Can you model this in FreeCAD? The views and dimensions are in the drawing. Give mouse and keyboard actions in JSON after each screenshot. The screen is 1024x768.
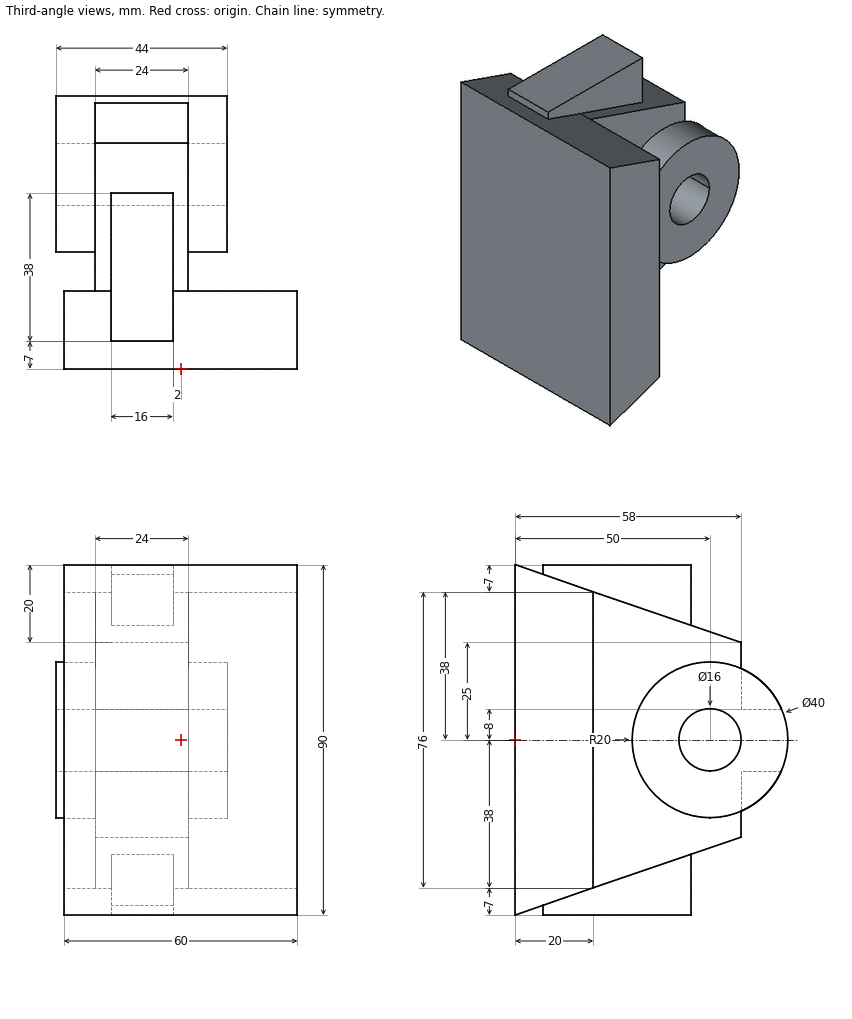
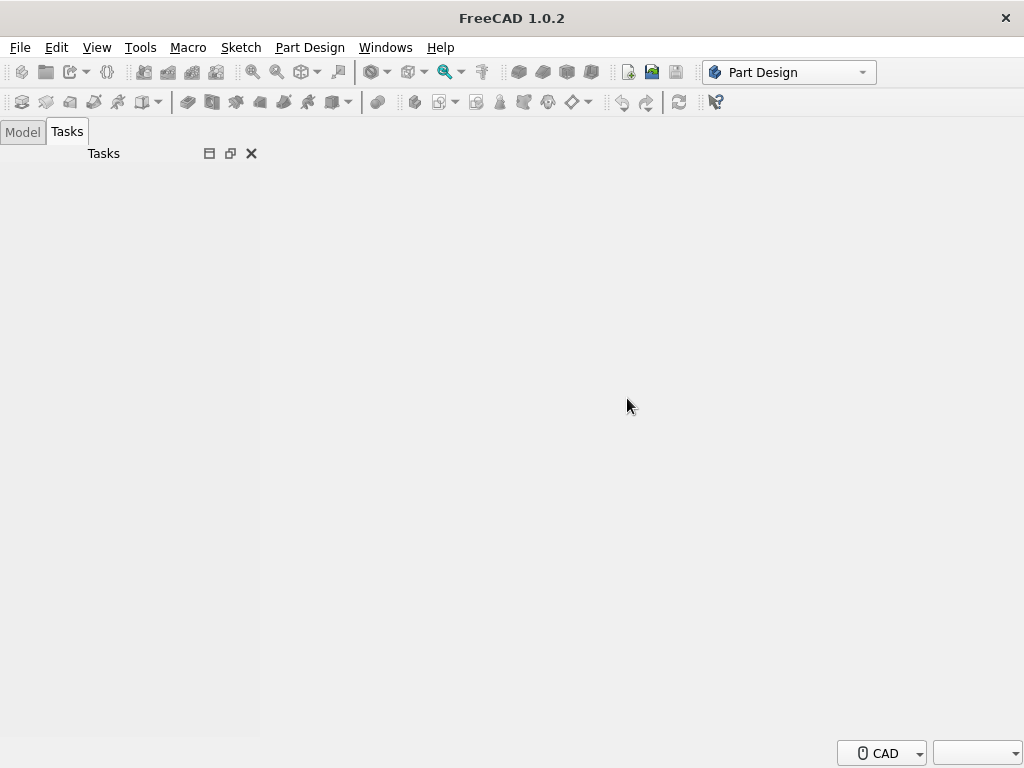
{"action": "left_click", "coordinate": [628, 72]}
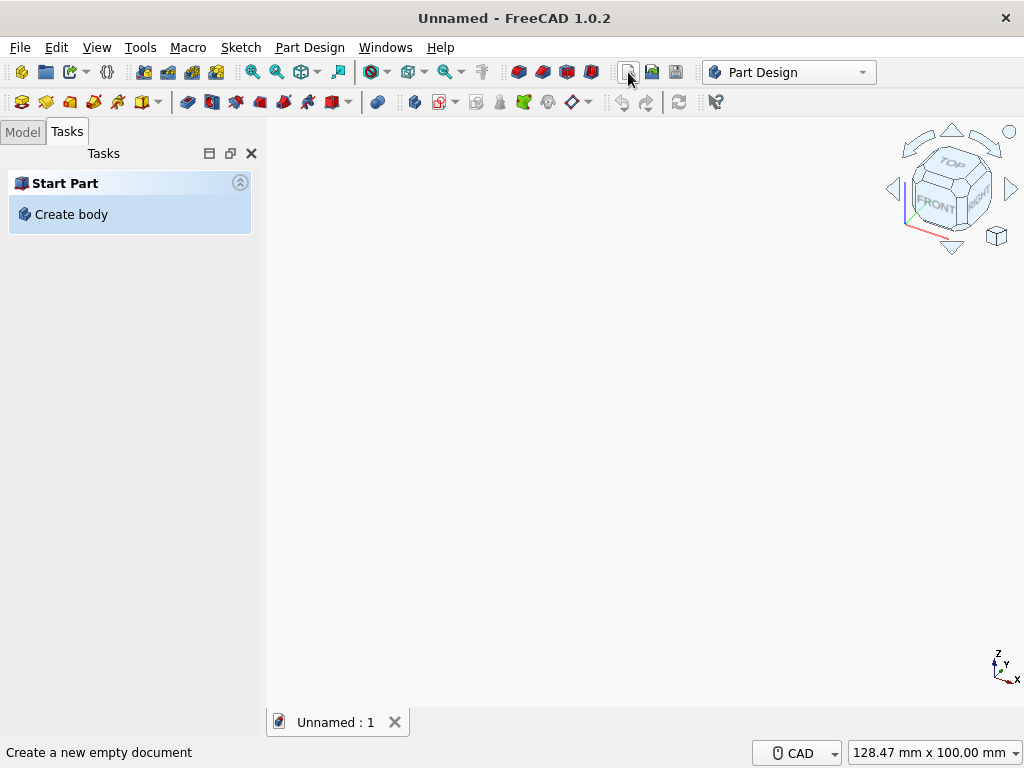
{"action": "left_click", "coordinate": [440, 102]}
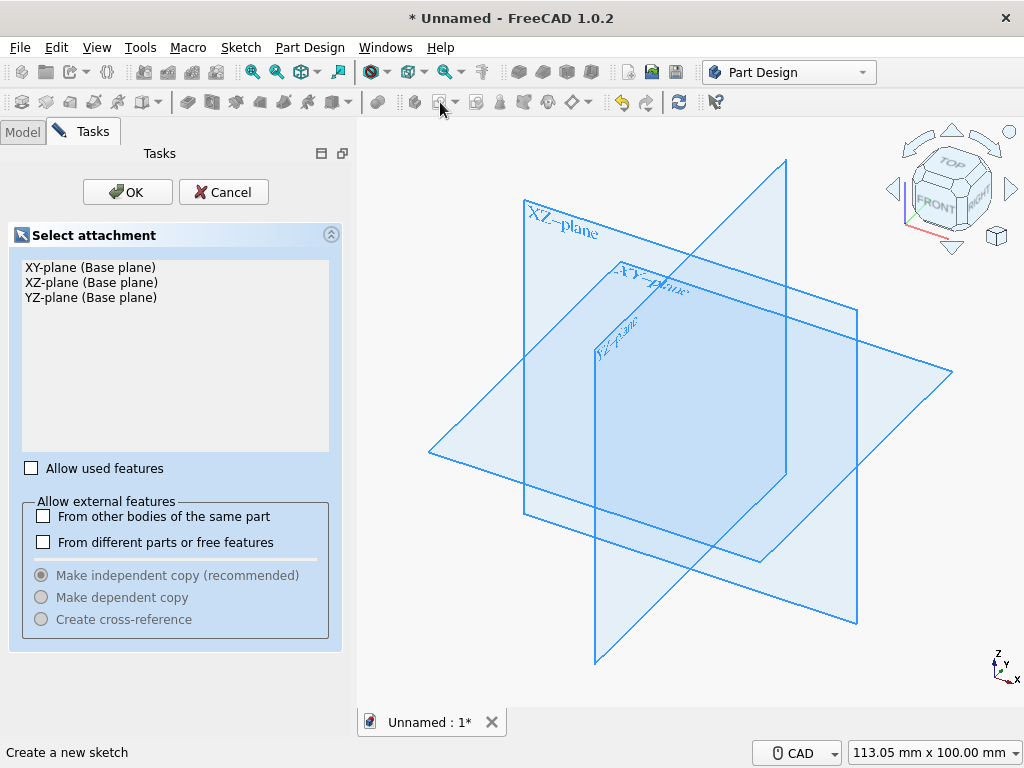
{"action": "left_click", "coordinate": [82, 282]}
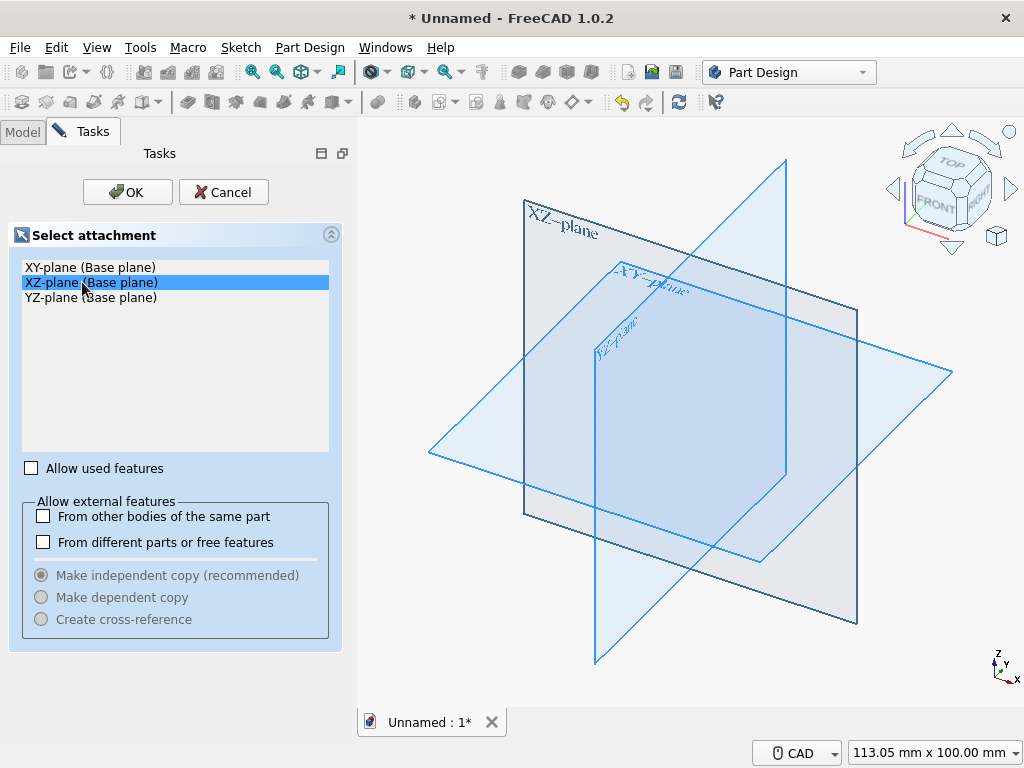
{"action": "left_click", "coordinate": [128, 192]}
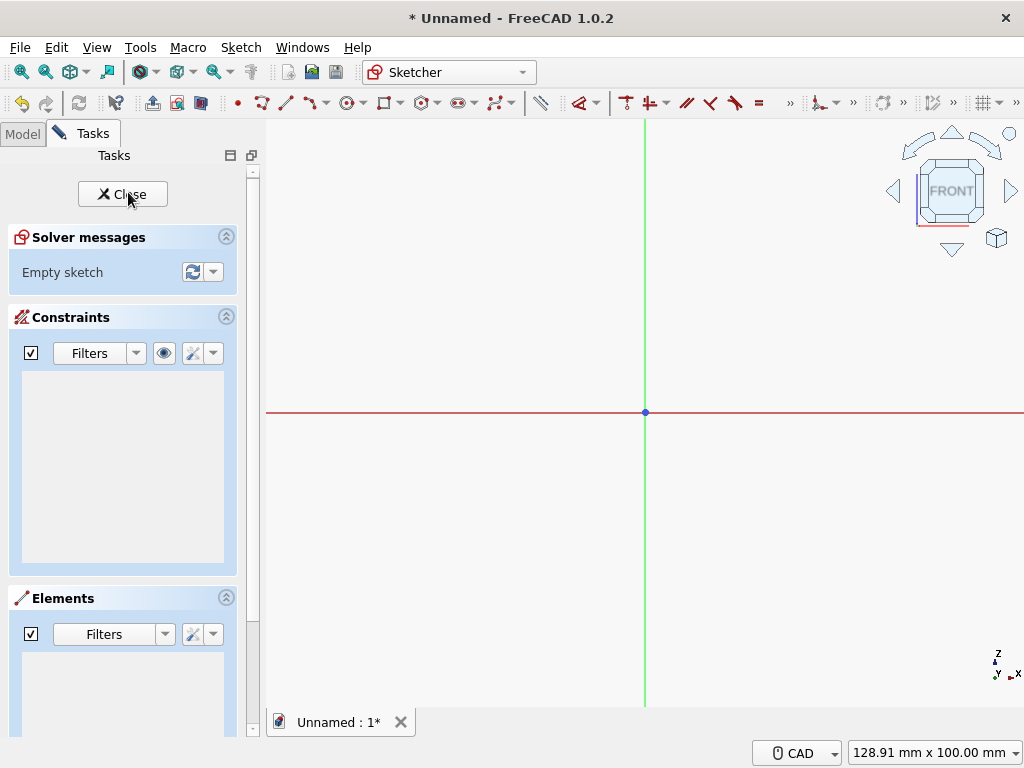
{"action": "scroll", "coordinate": [437, 413], "scroll_direction": "down", "scroll_amount": 2}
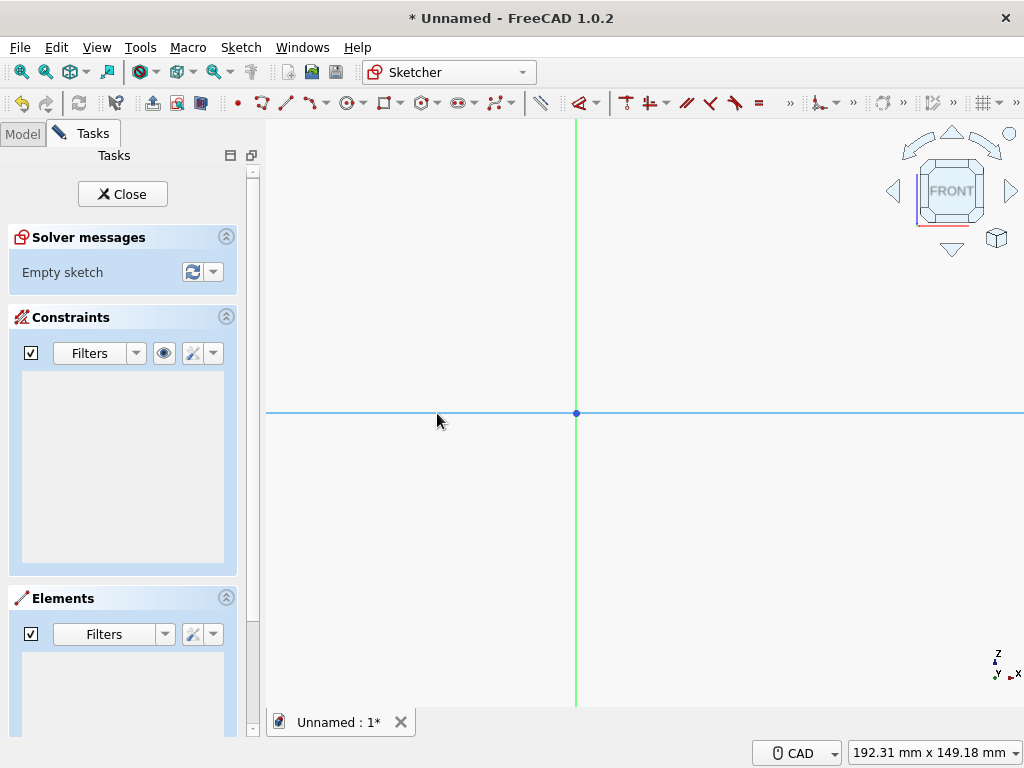
{"action": "key", "text": "g v"}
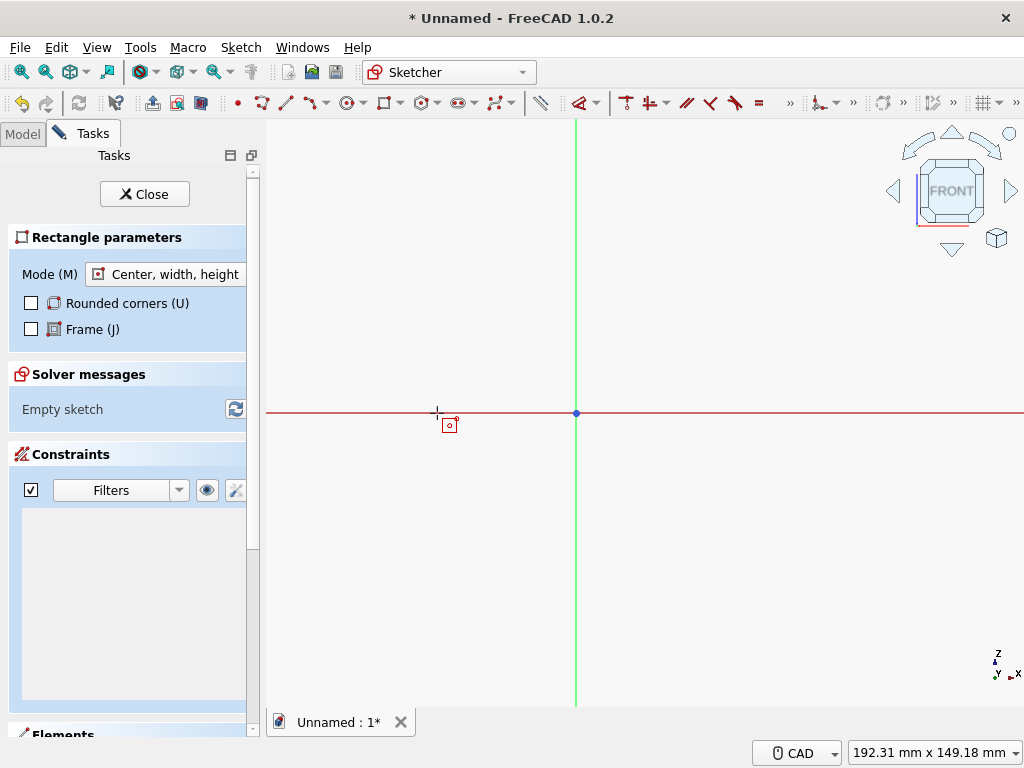
{"action": "left_click", "coordinate": [577, 413]}
{"action": "mouse_move", "coordinate": [695, 236]}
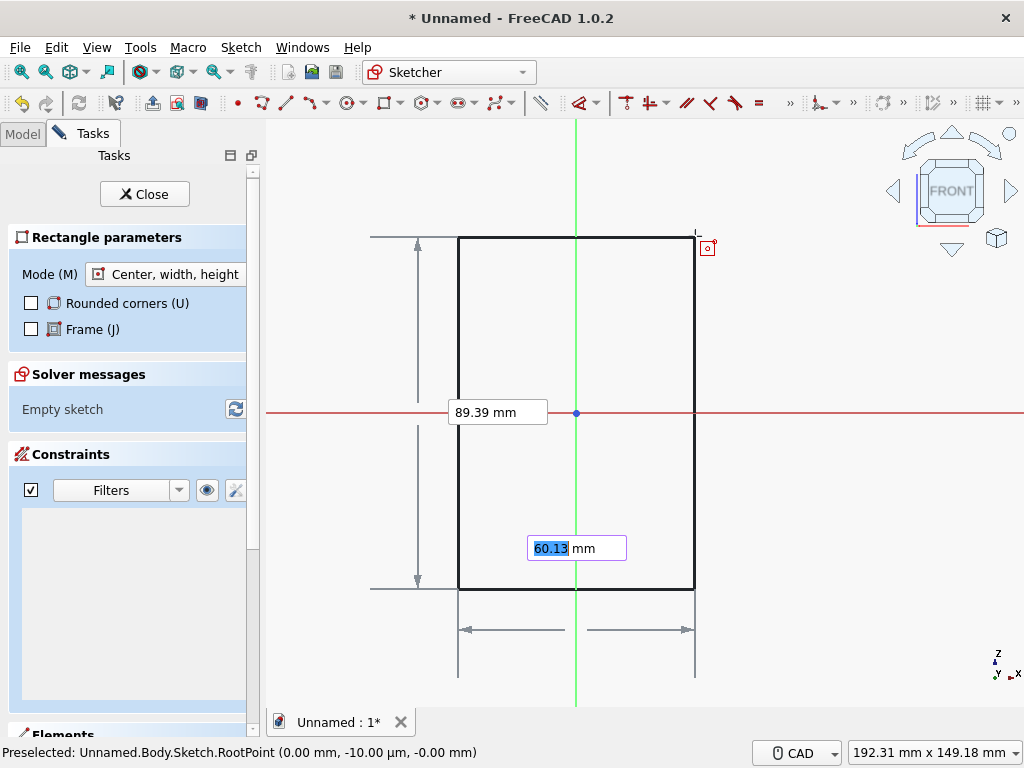
{"action": "type", "text": "60"}
{"action": "key", "text": "Tab"}
{"action": "type", "text": "90"}
{"action": "key", "text": "Return"}
{"action": "key", "text": "Escape"}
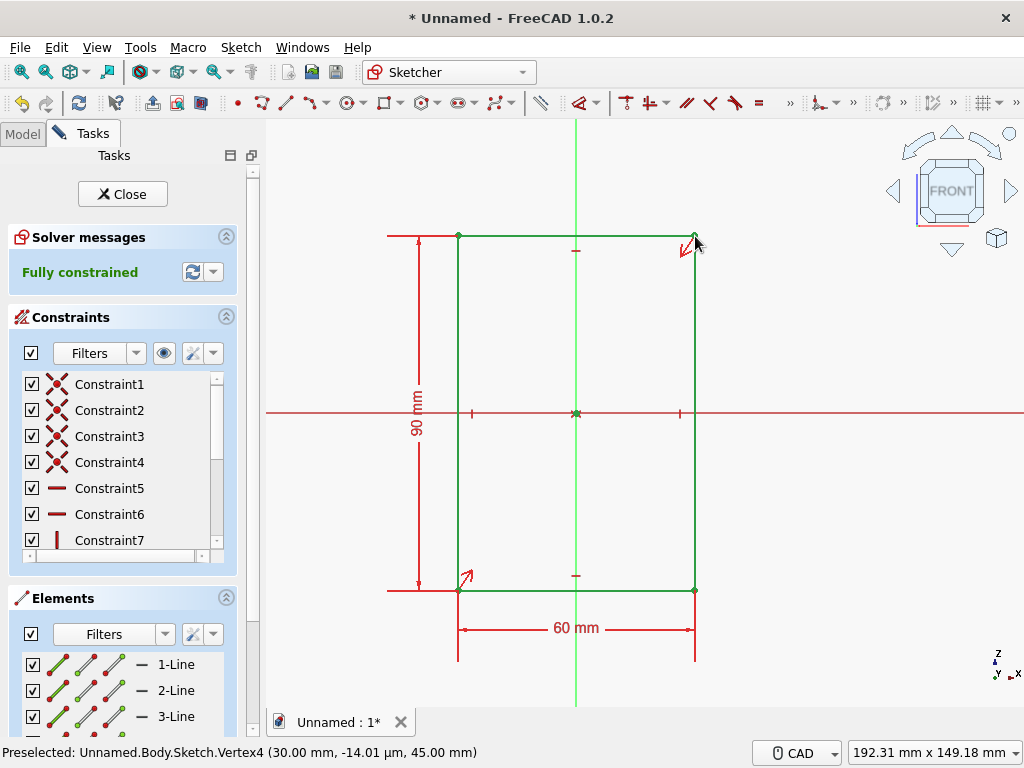
{"action": "left_click", "coordinate": [123, 194]}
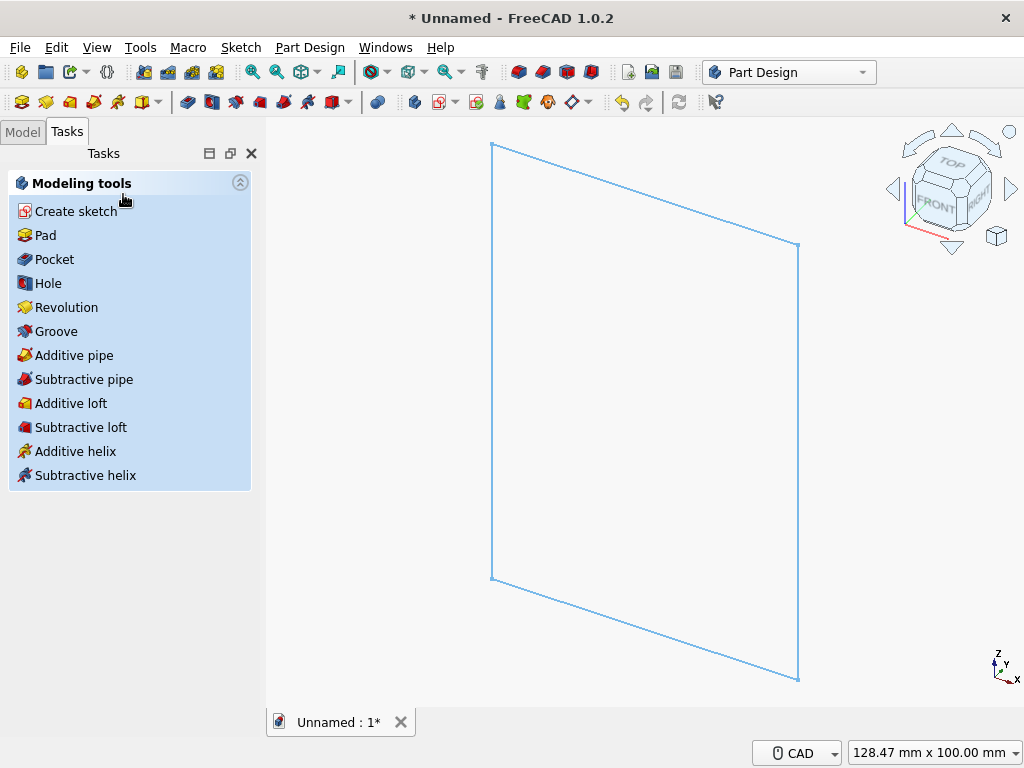
{"action": "left_click", "coordinate": [22, 102]}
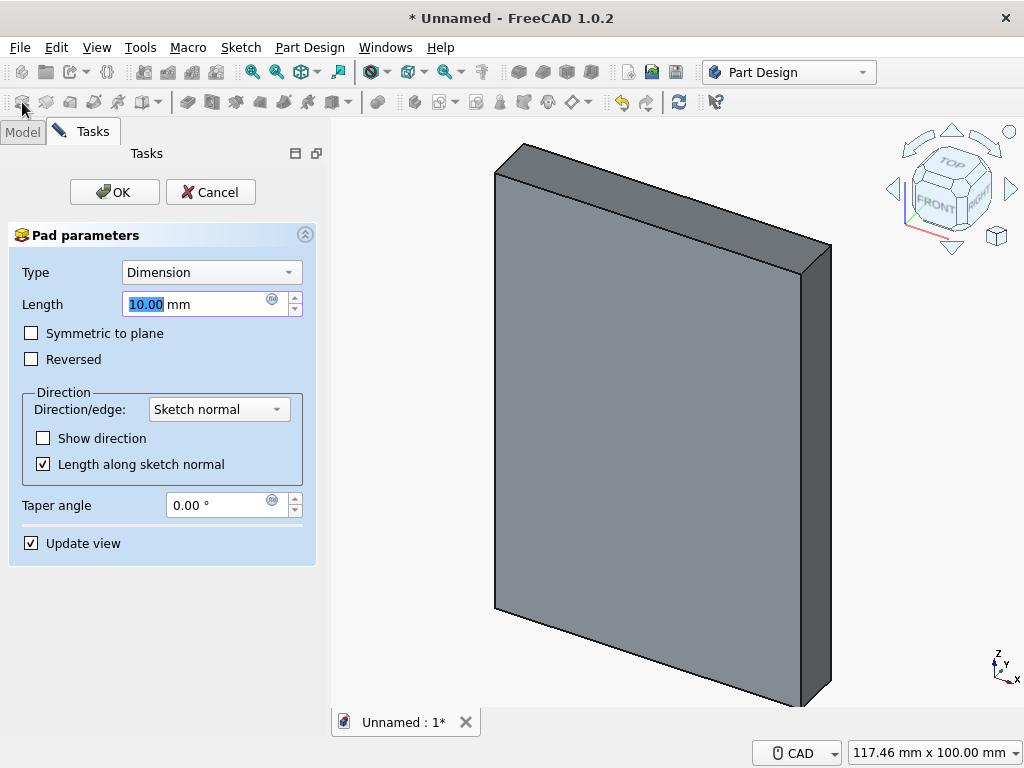
{"action": "type", "text": "20"}
{"action": "key", "text": "Tab"}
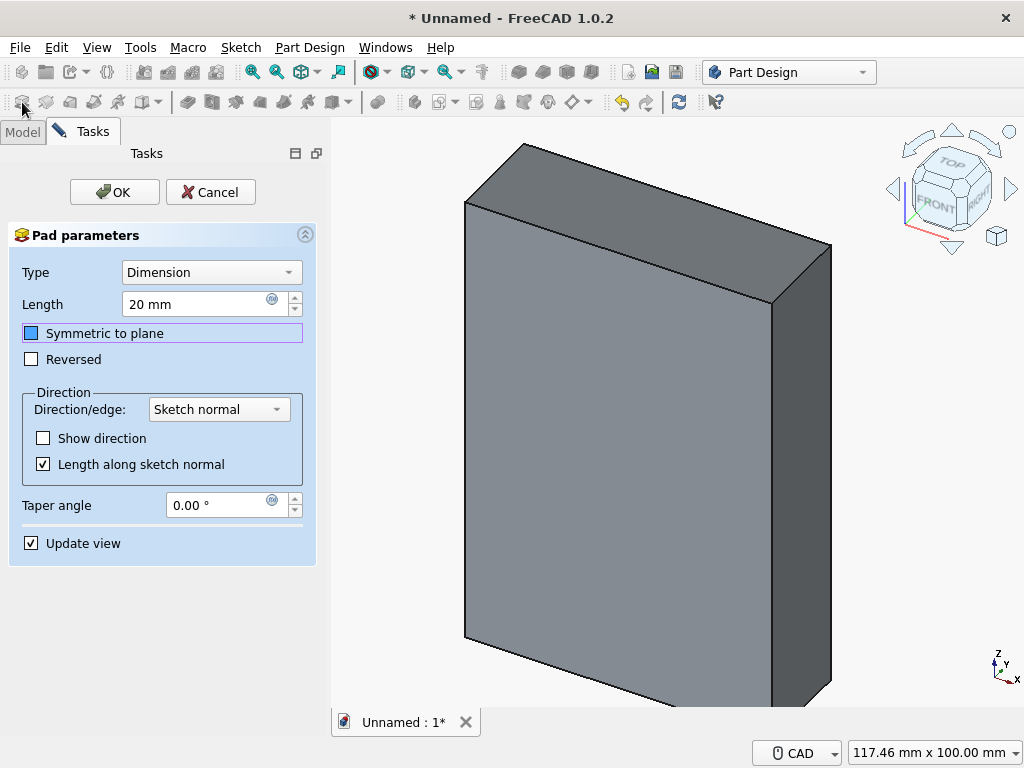
{"action": "left_click", "coordinate": [30, 359]}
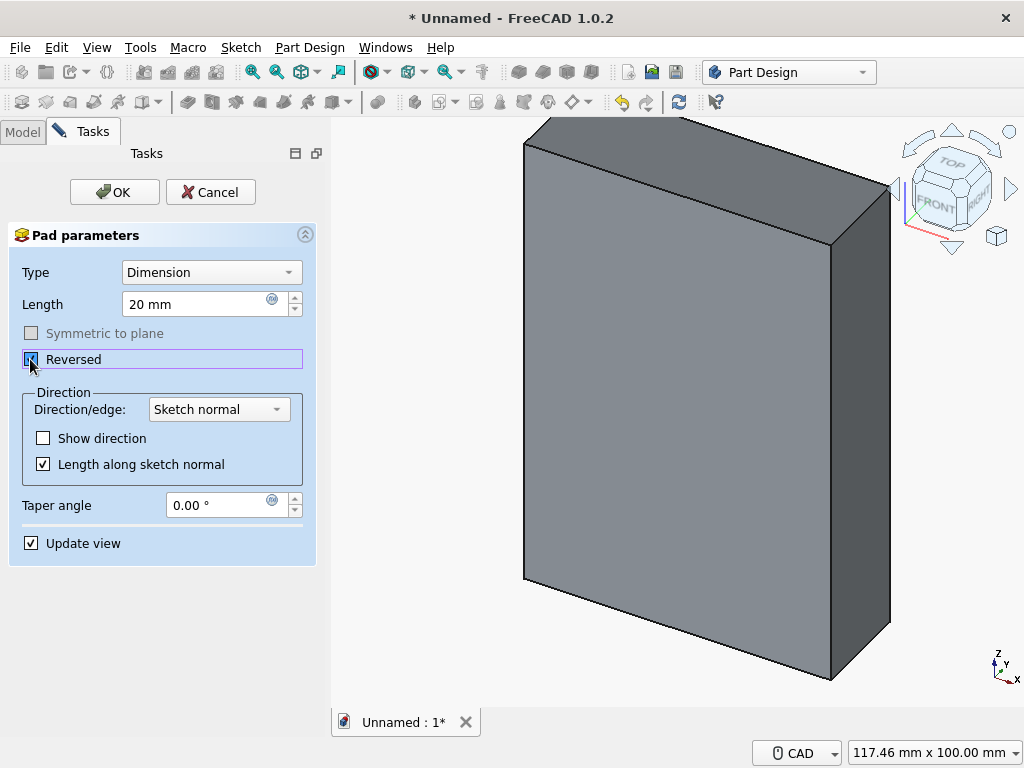
{"action": "left_click", "coordinate": [115, 192]}